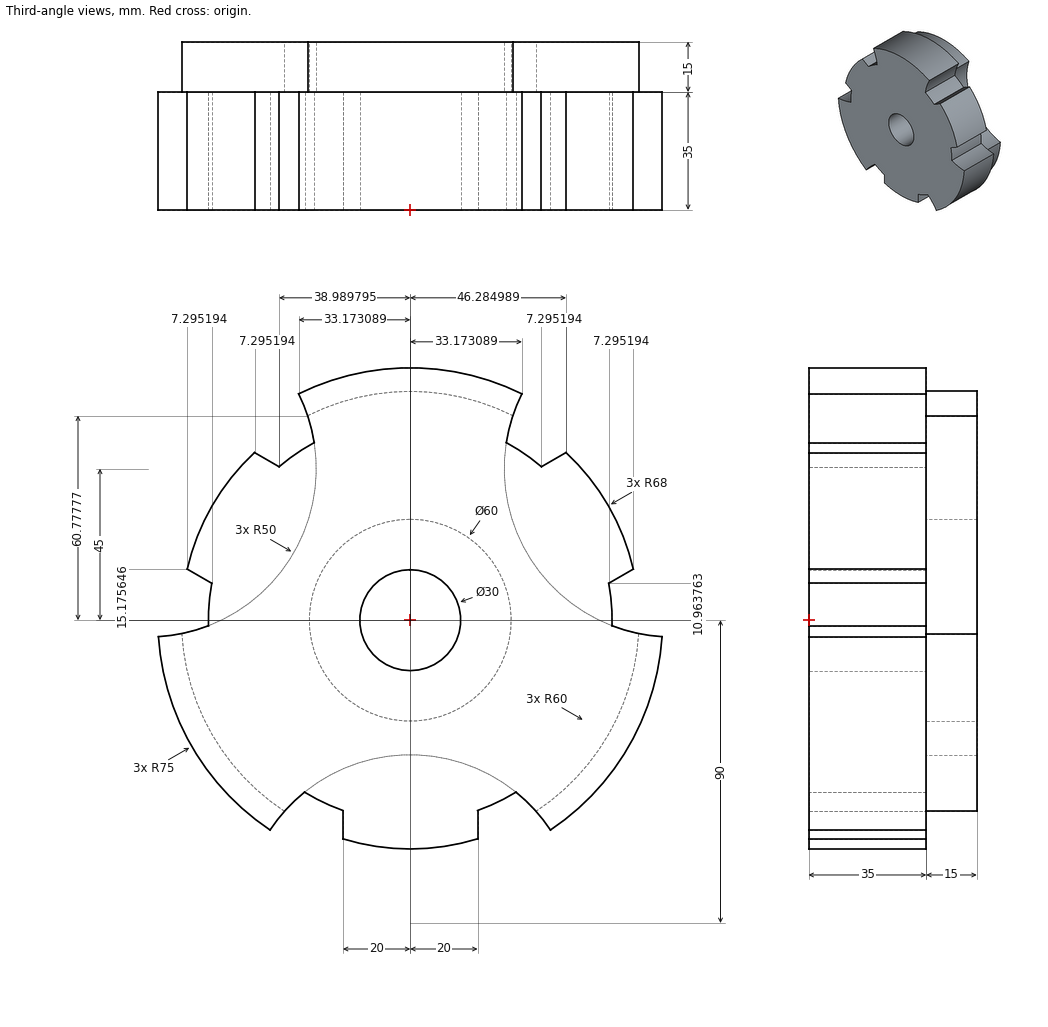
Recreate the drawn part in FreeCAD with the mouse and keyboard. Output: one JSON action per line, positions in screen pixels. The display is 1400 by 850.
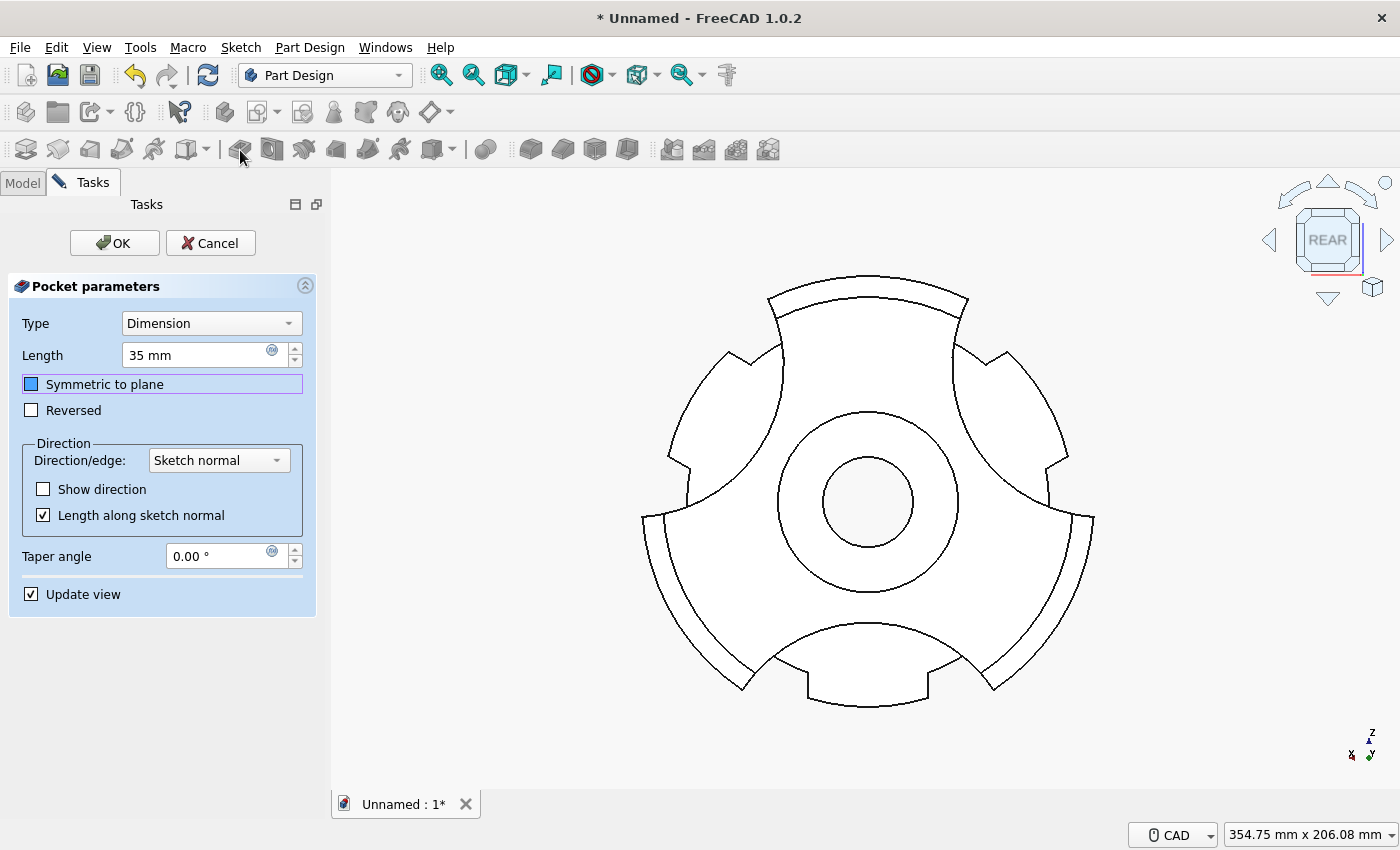
{"action": "left_click", "coordinate": [115, 243]}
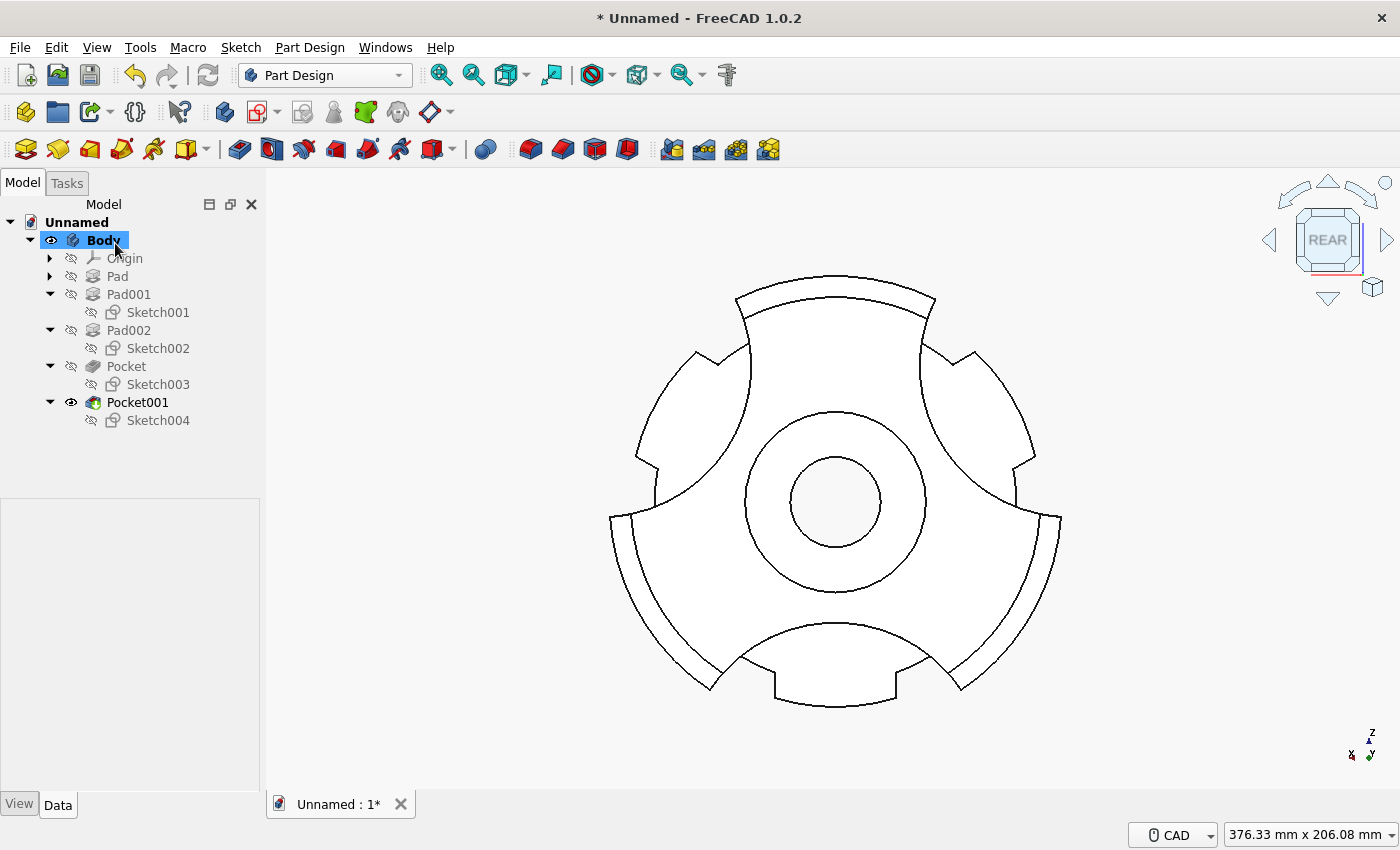
{"action": "key", "text": "0"}